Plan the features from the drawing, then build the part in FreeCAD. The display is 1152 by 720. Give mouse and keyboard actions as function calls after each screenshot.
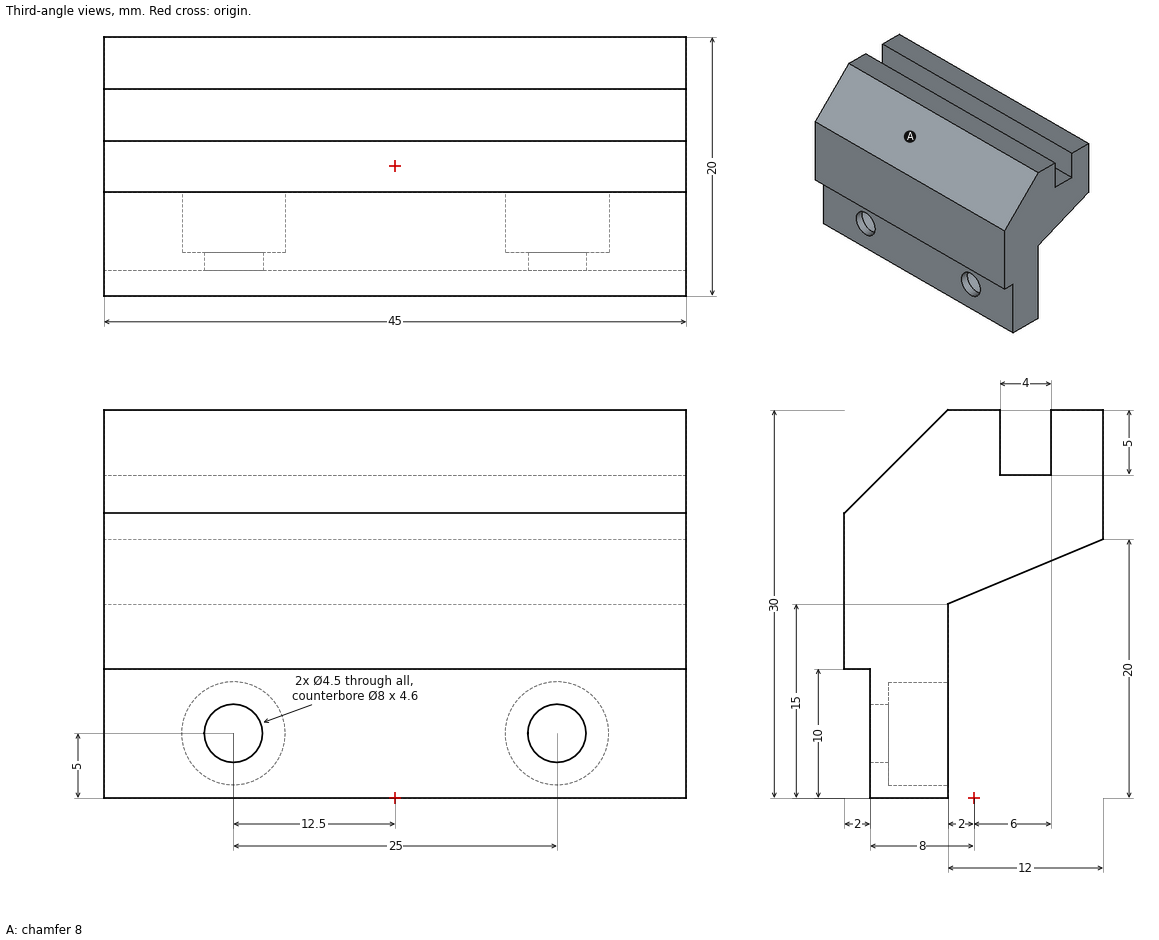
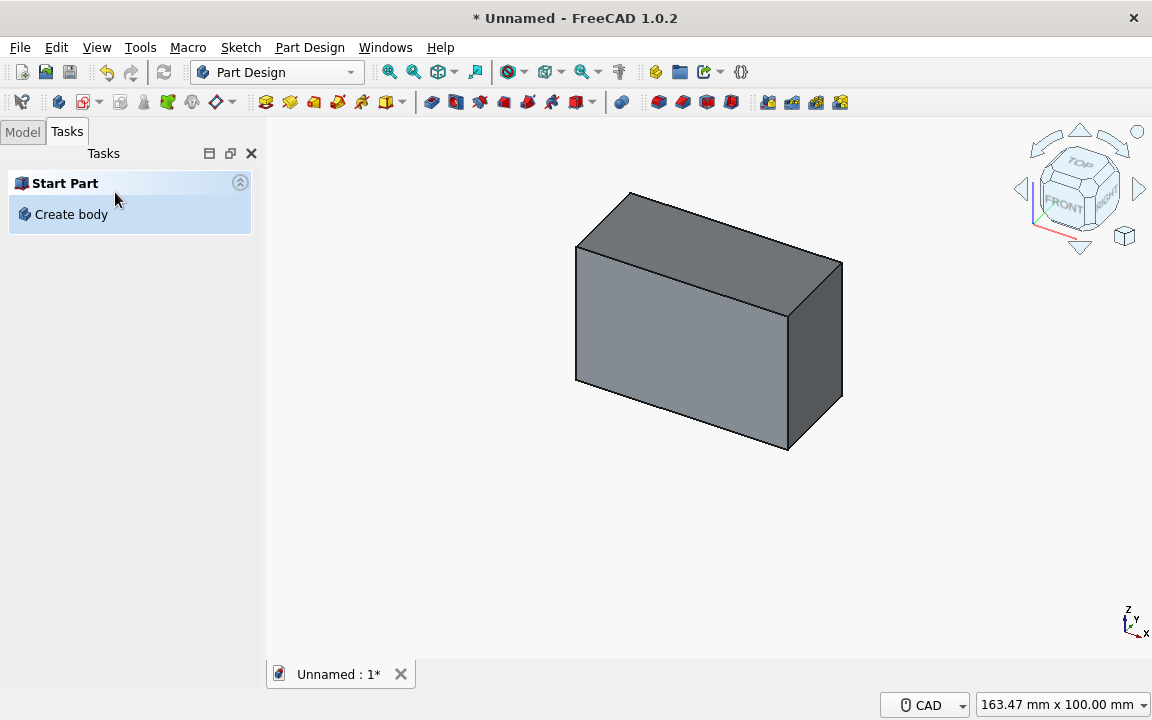
key(6)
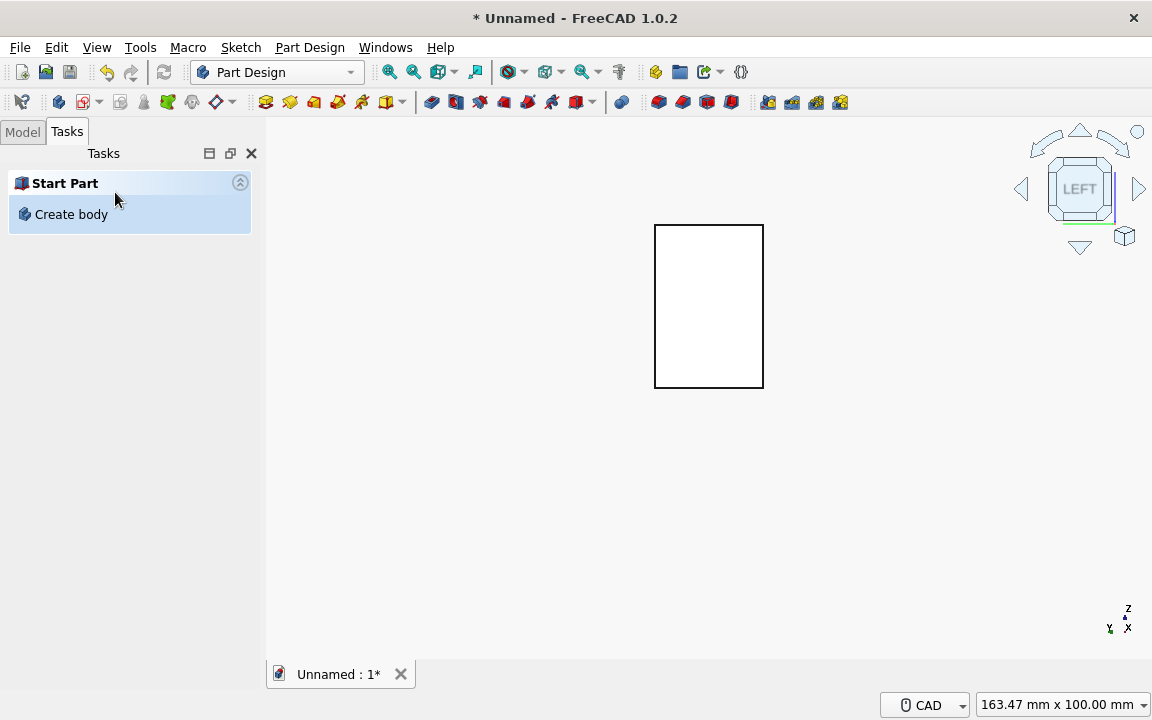
key(v)
key(f)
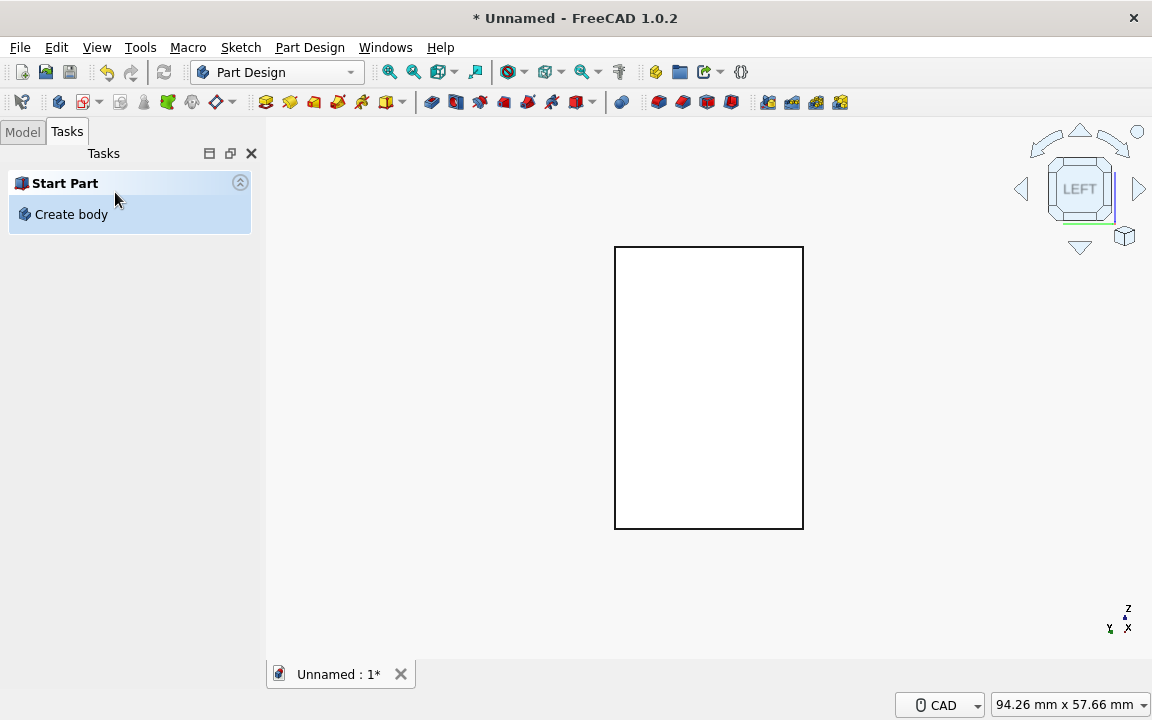
click(709, 347)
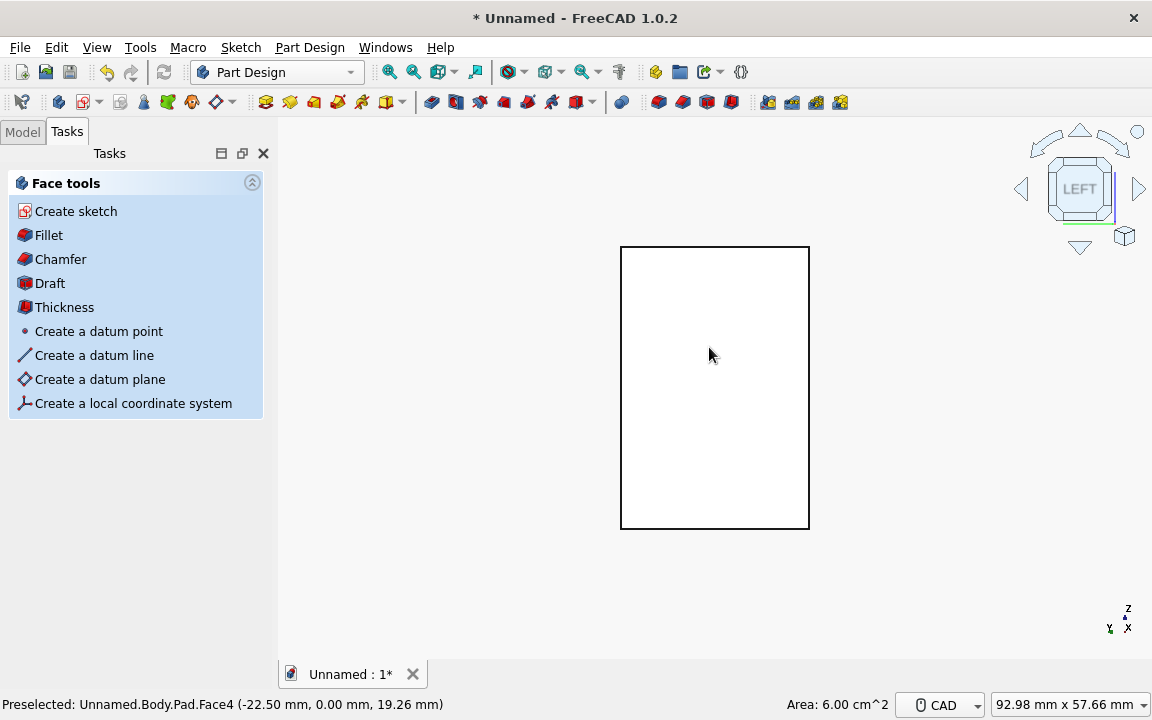
click(84, 102)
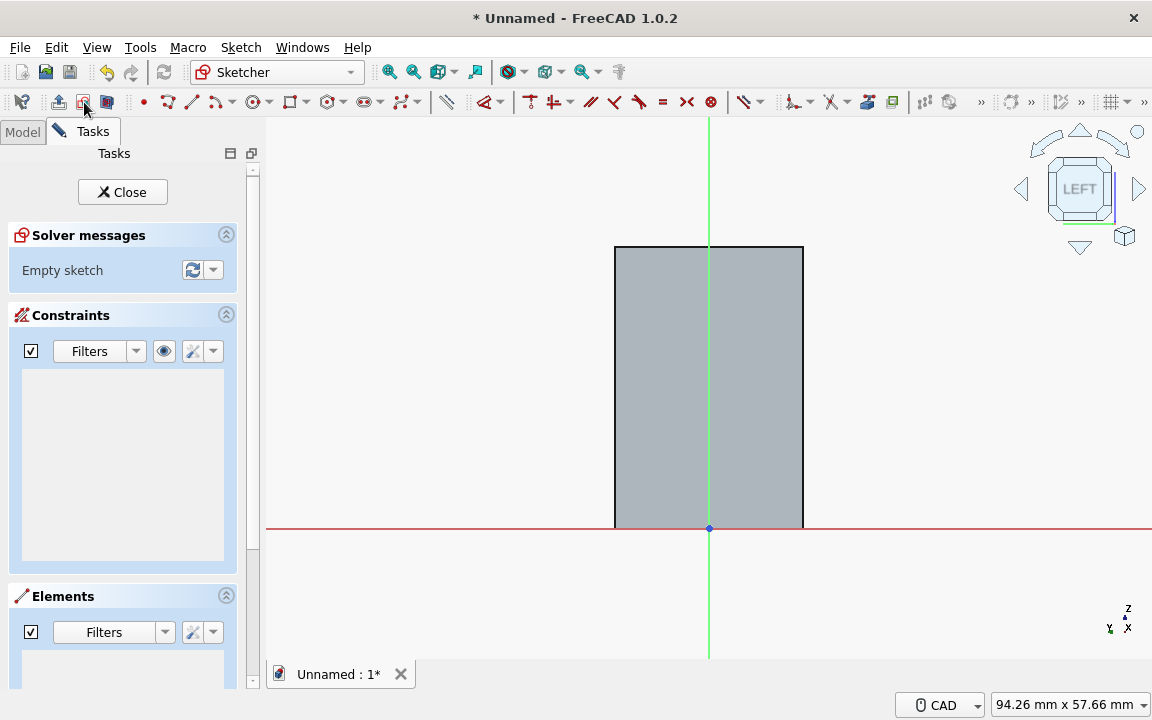
click(168, 102)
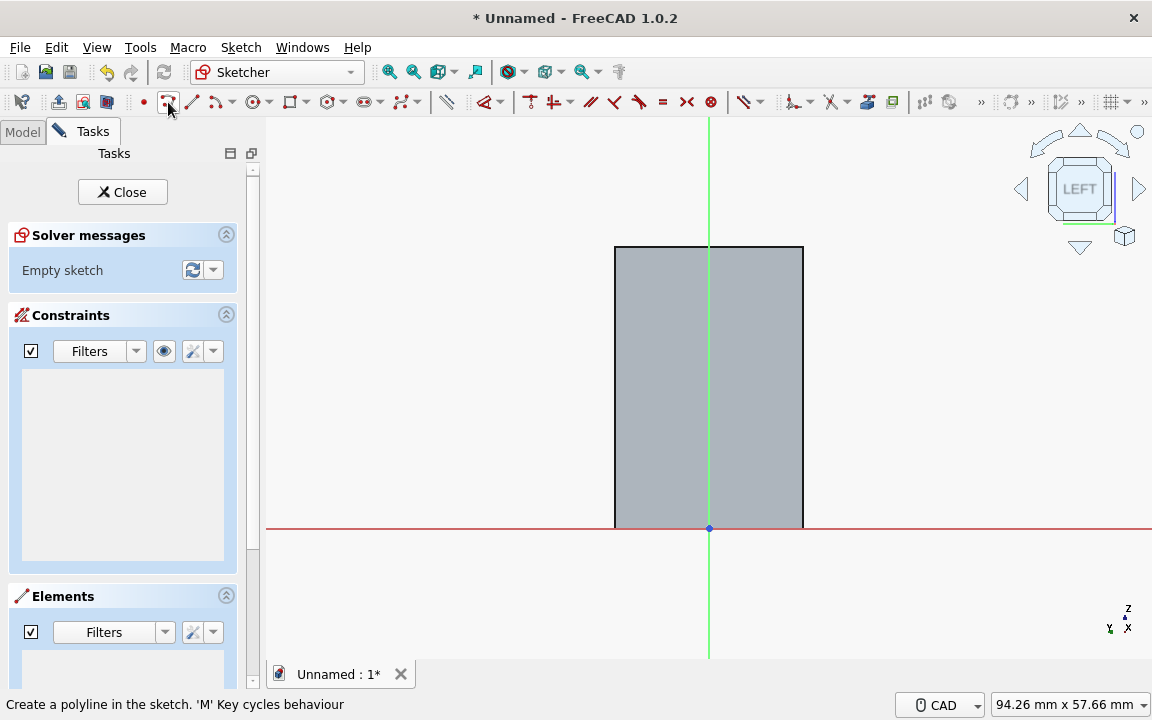
click(728, 529)
click(728, 388)
click(615, 341)
click(615, 520)
click(728, 529)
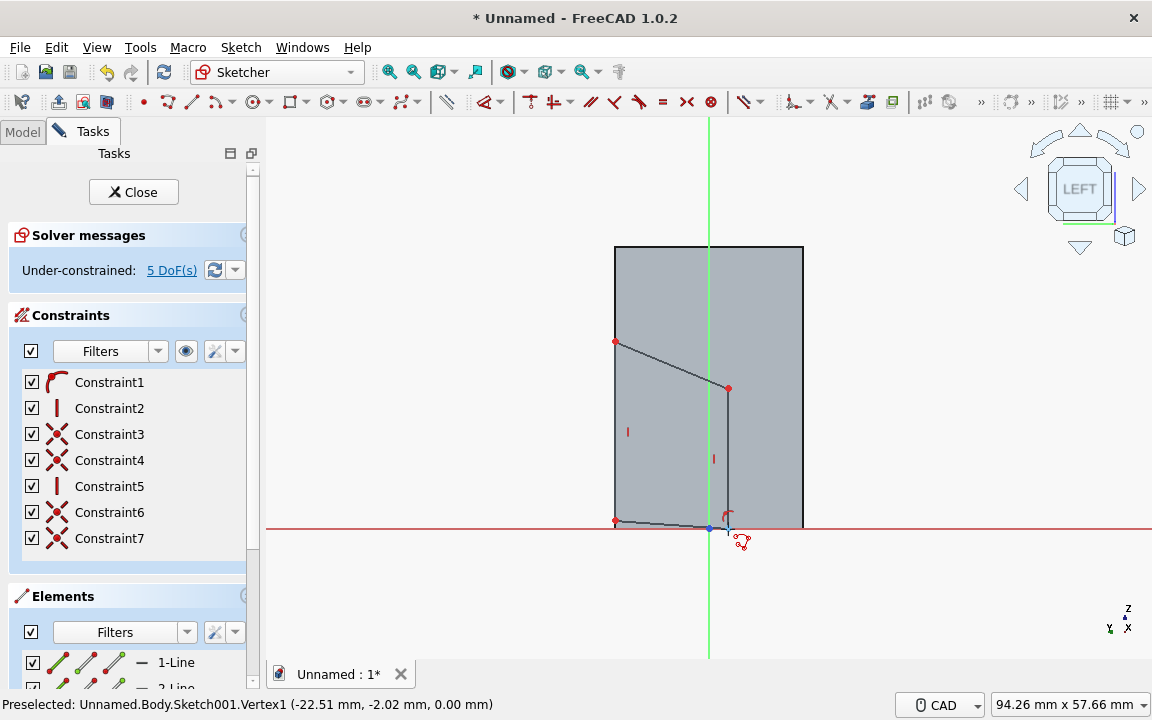
click(290, 102)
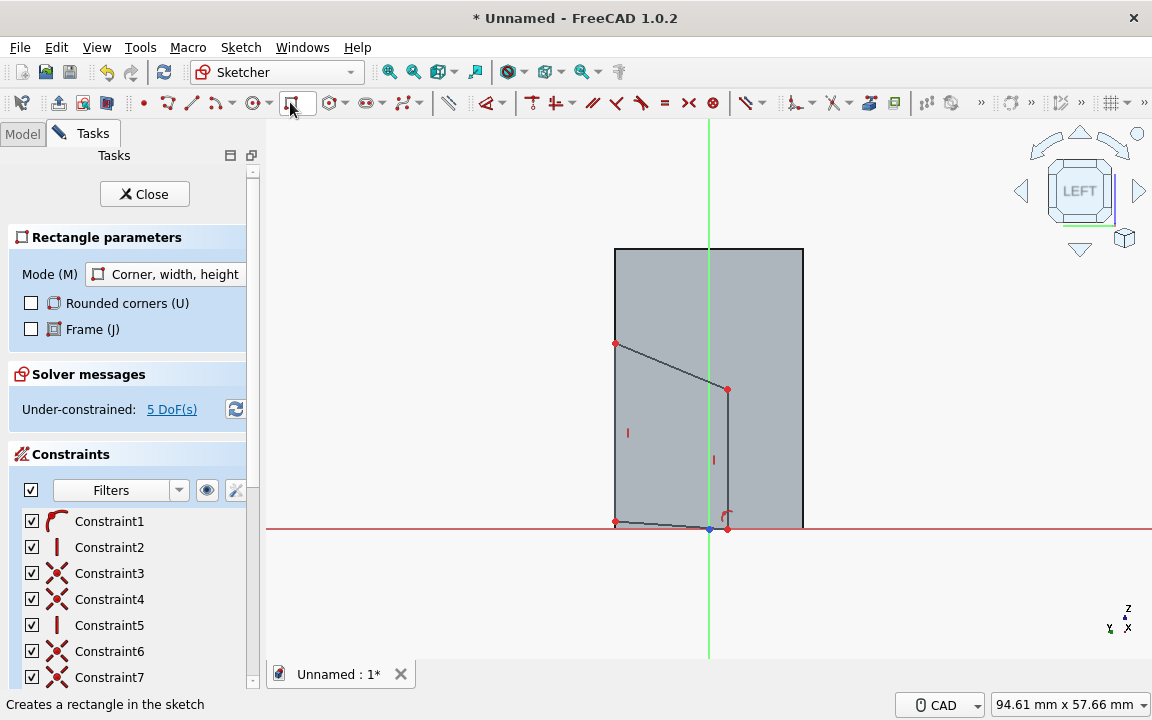
click(653, 249)
move(690, 295)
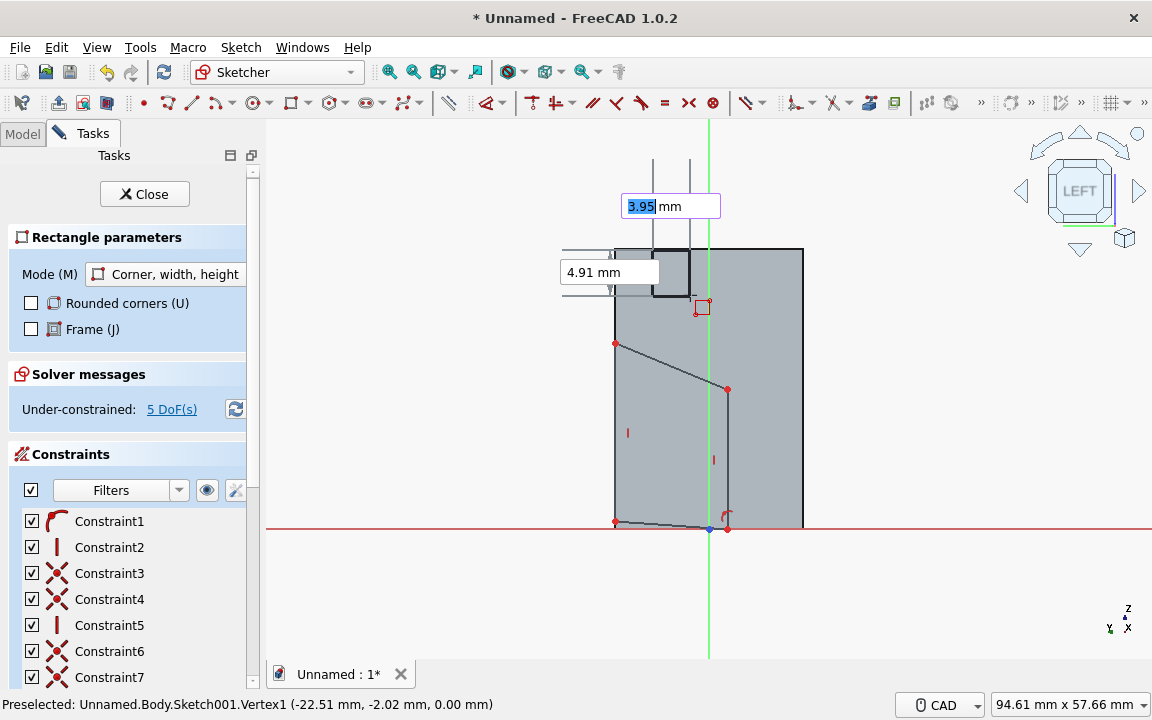
text(4)
key(Tab)
text(5)
key(Return)
key(Escape)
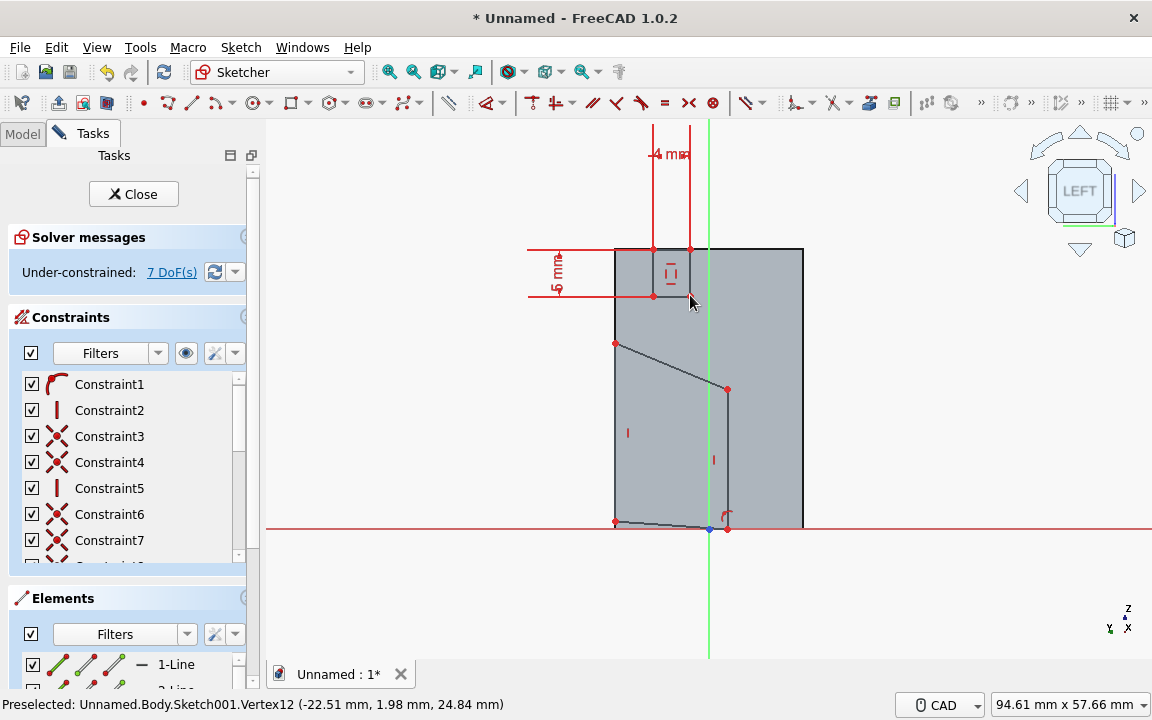
click(694, 527)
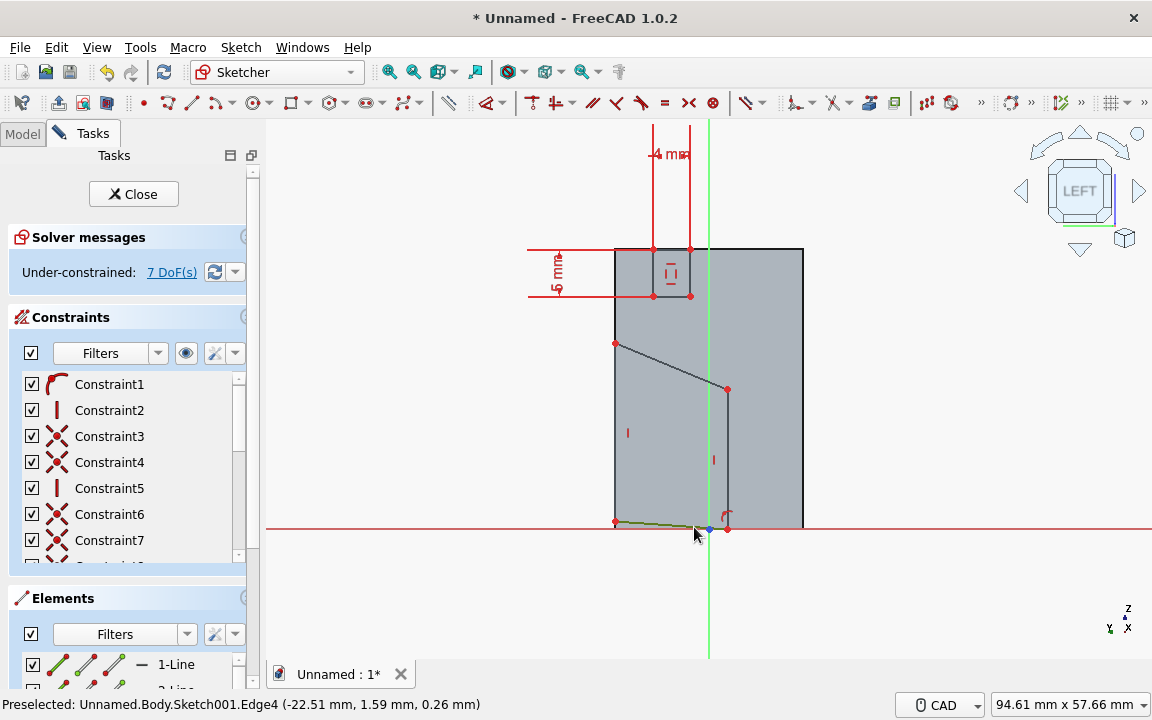
key(h)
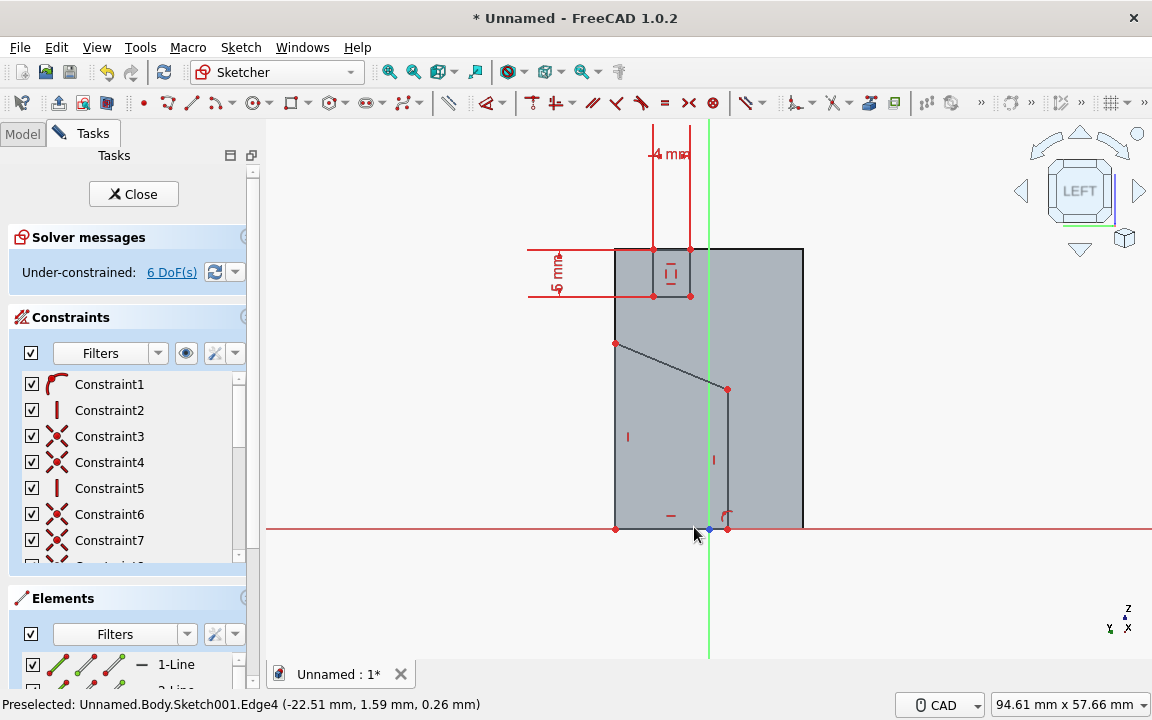
click(728, 488)